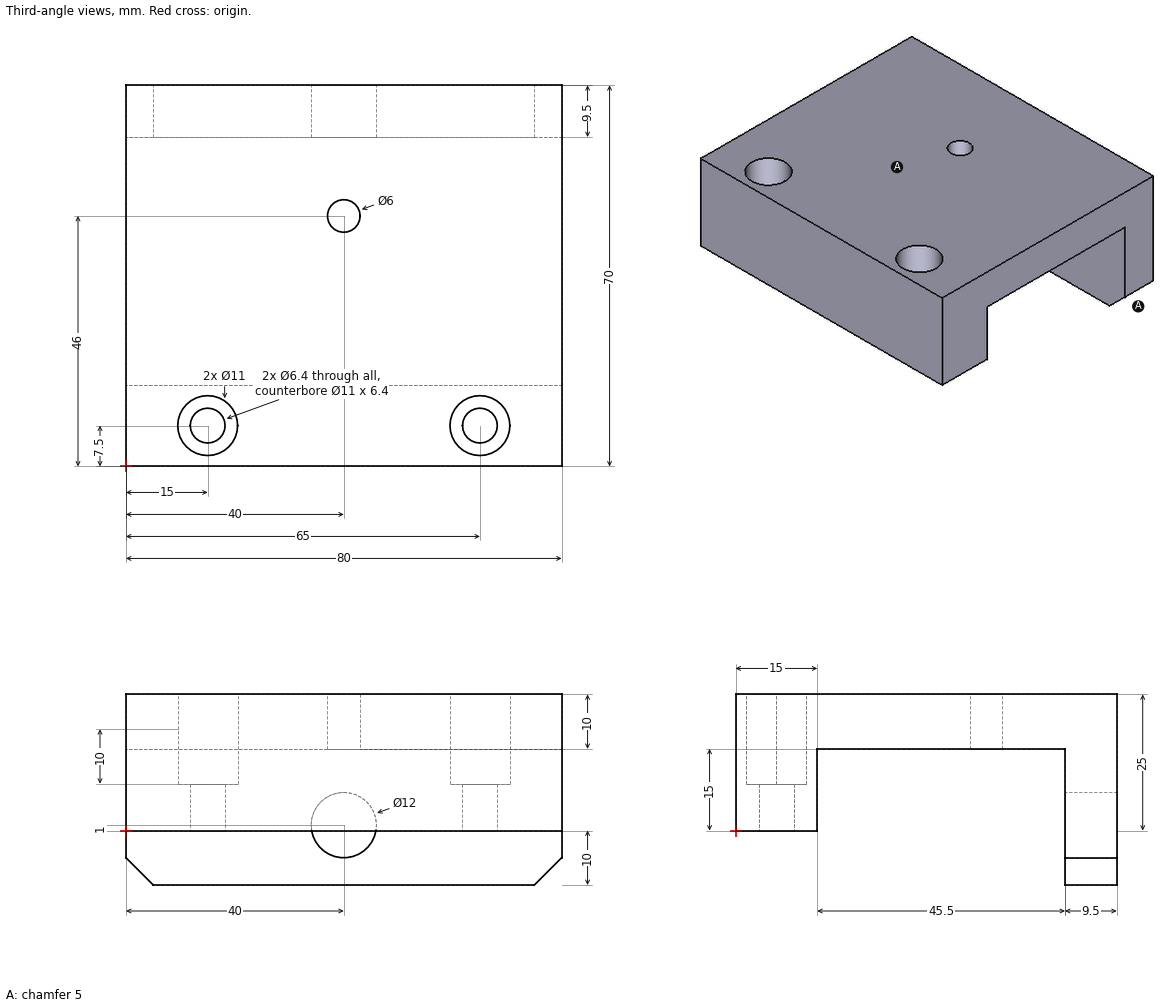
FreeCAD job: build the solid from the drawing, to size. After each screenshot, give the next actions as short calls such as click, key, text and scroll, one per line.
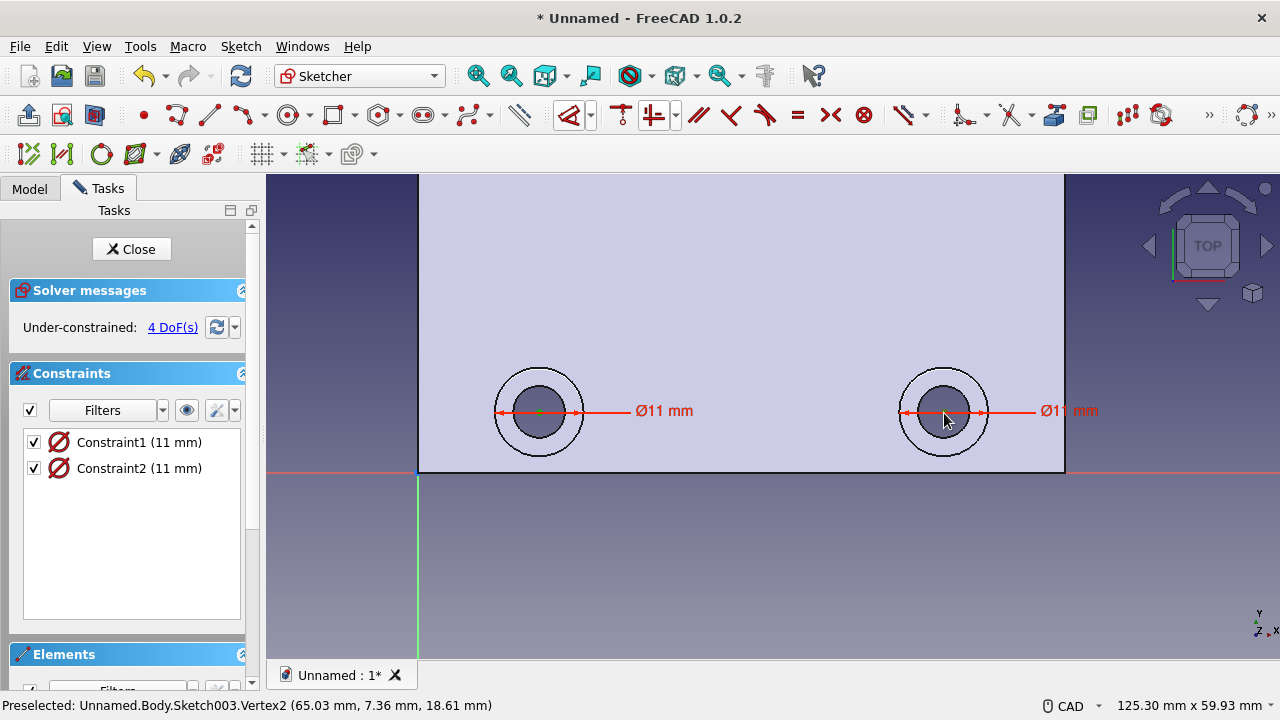
click(676, 116)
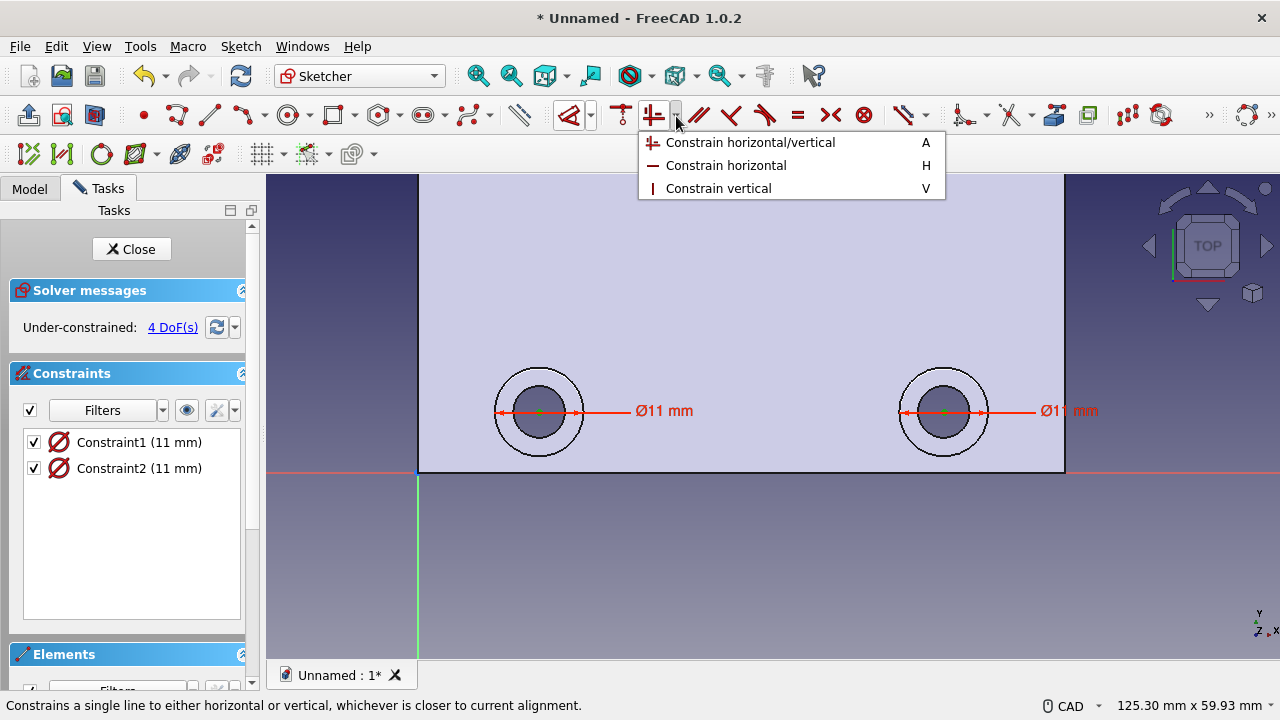
click(792, 166)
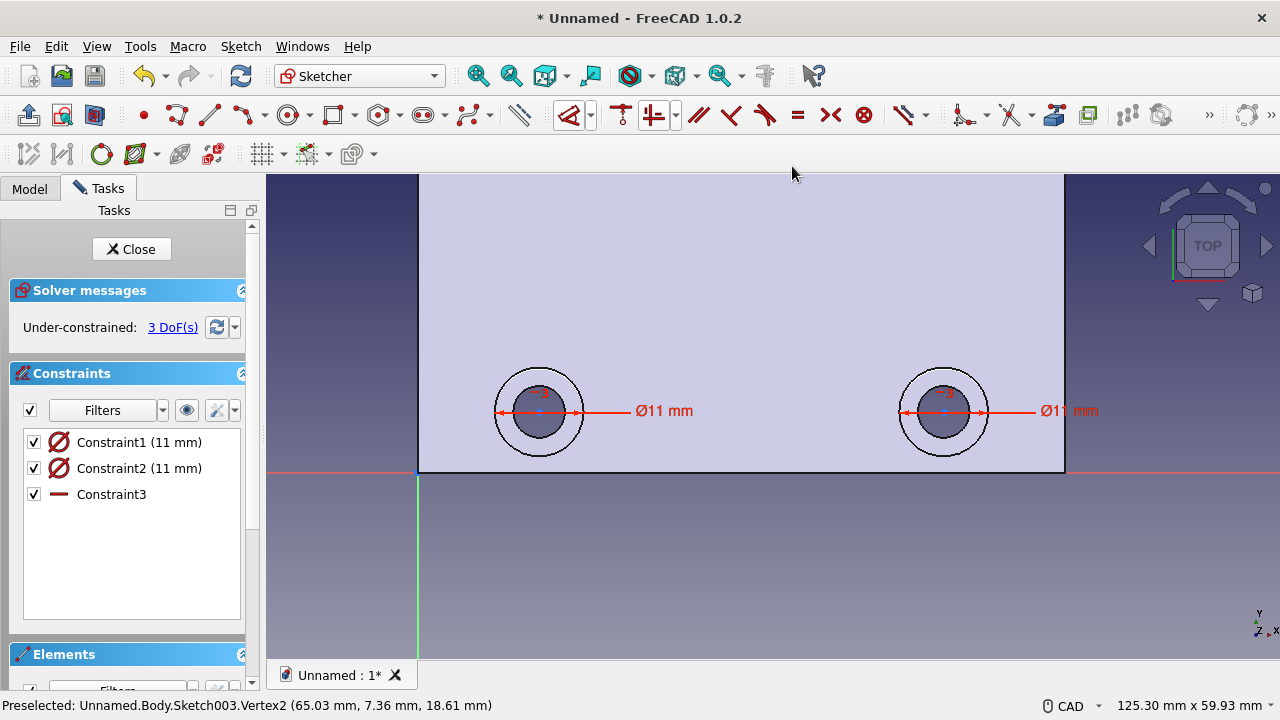
click(539, 413)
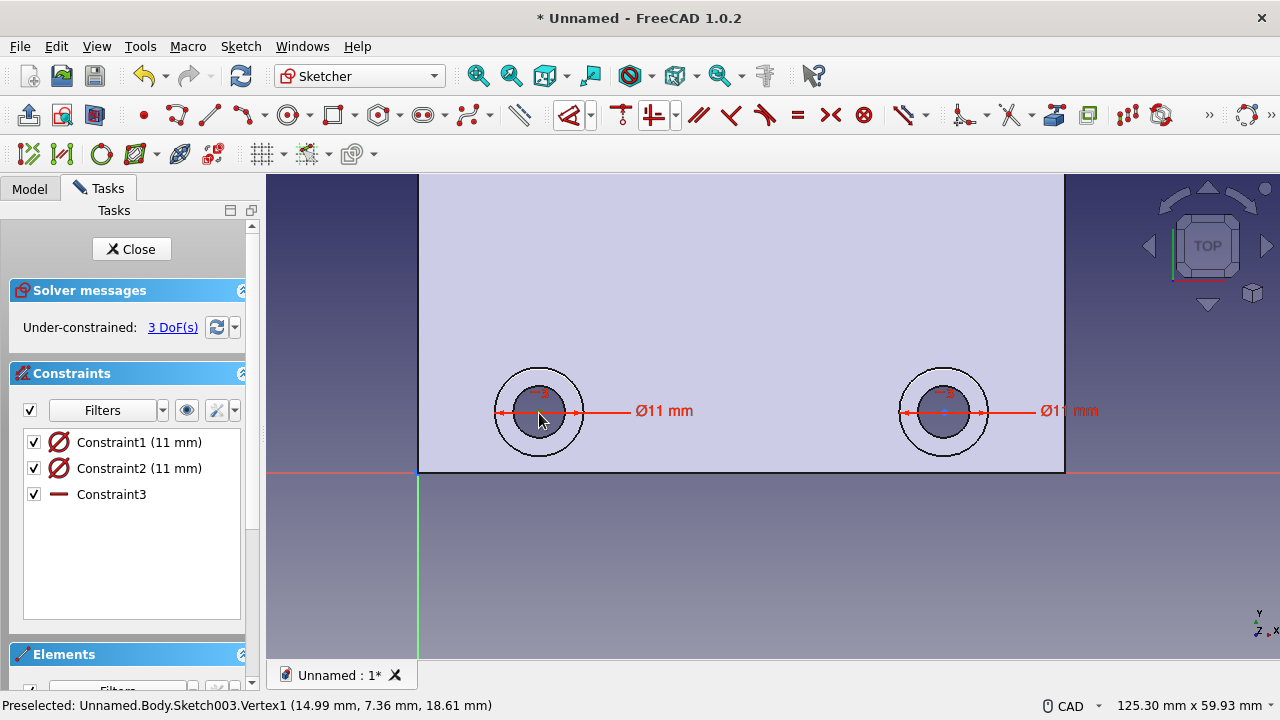
click(590, 116)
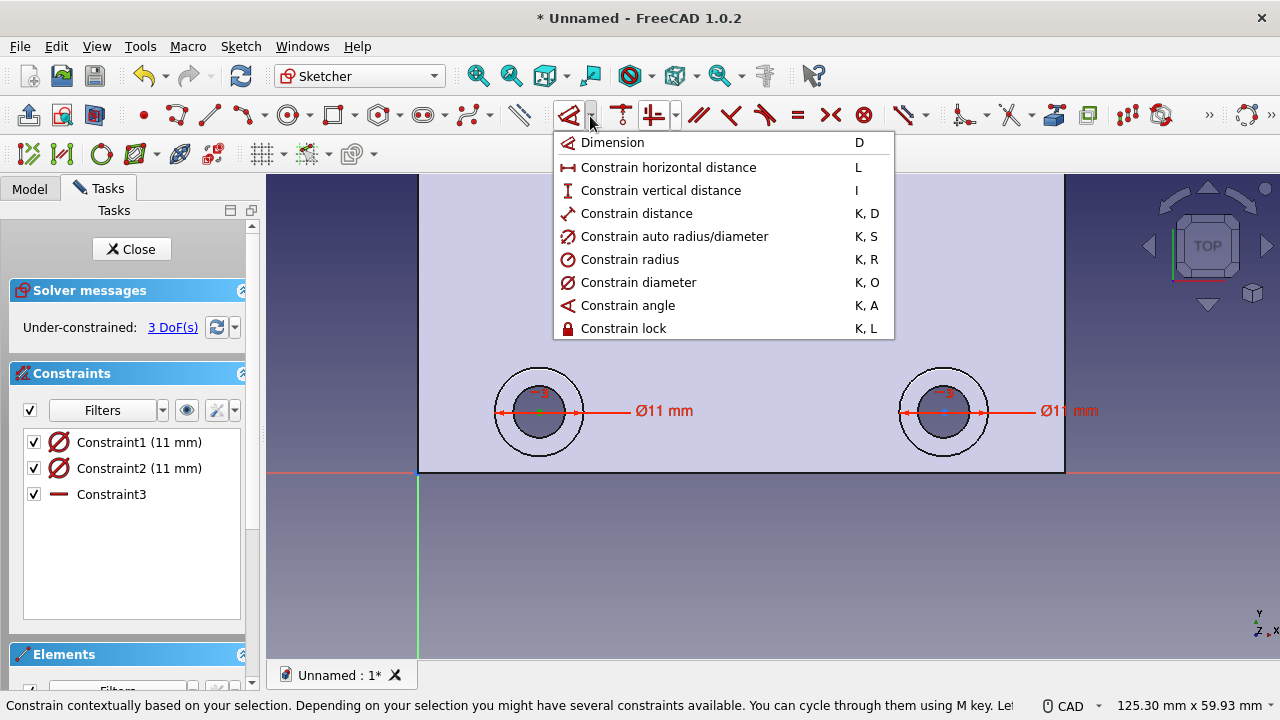
click(724, 168)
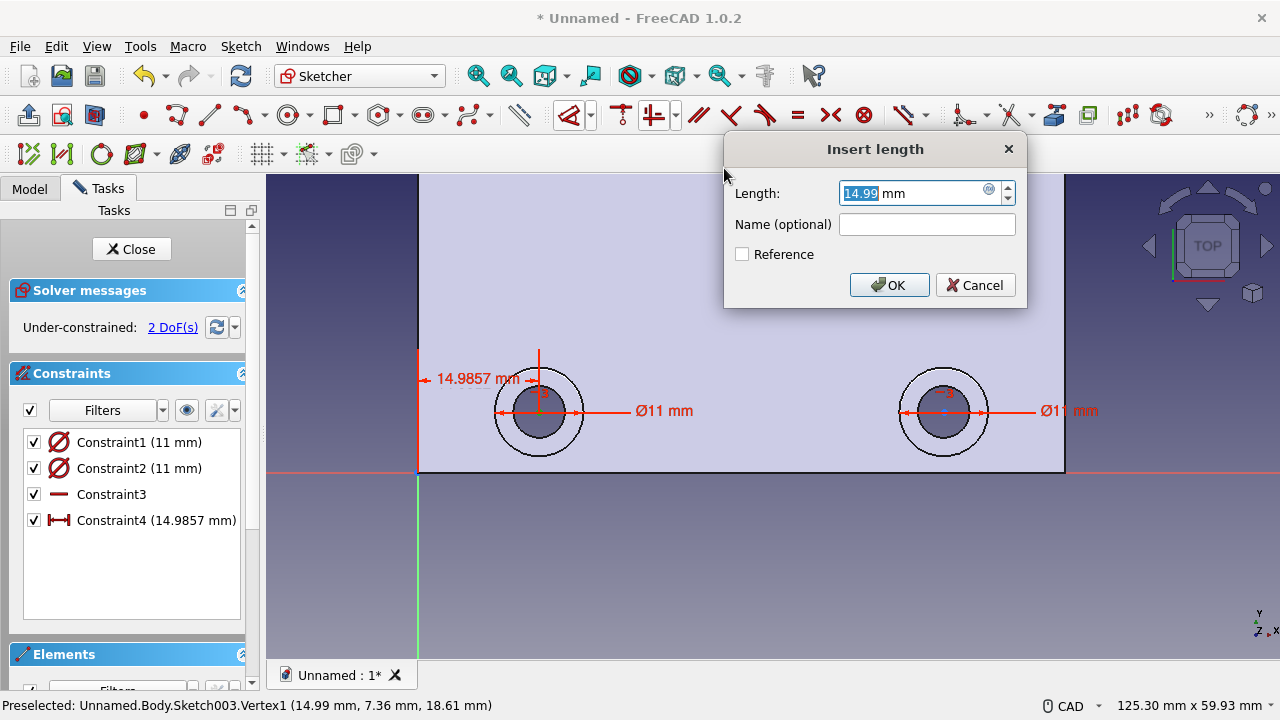
text(15)
key(Return)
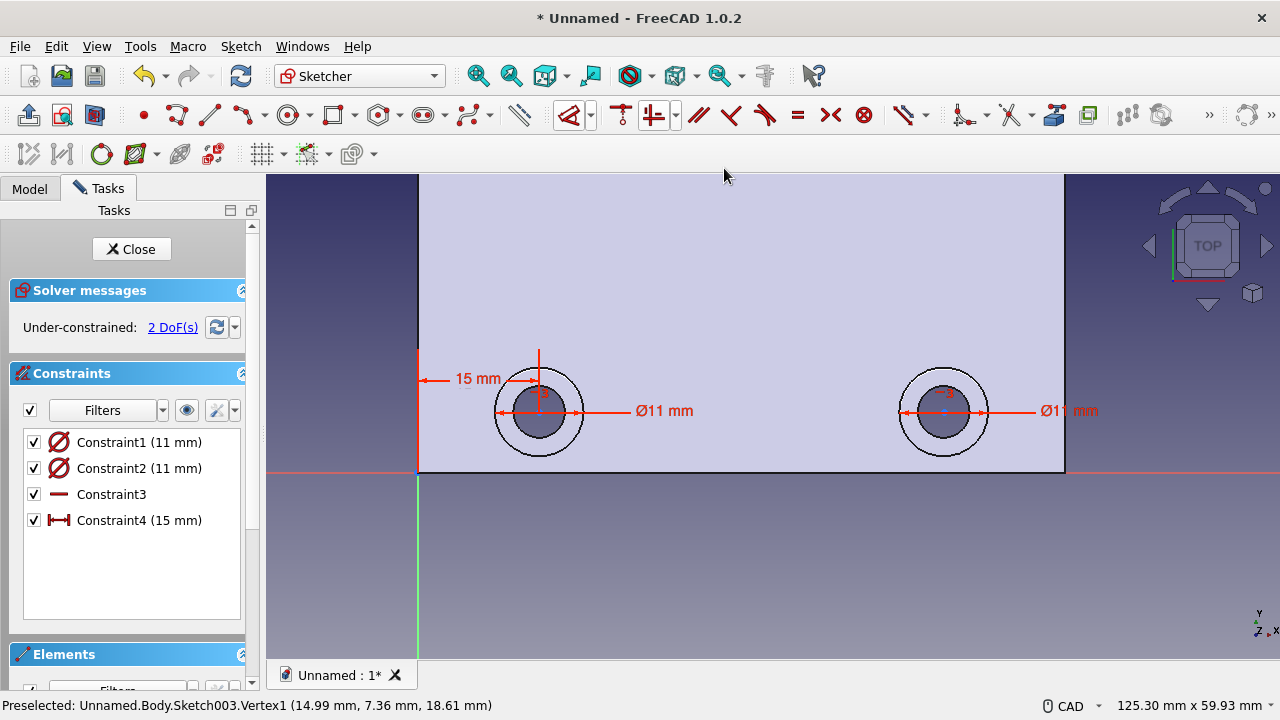
click(944, 413)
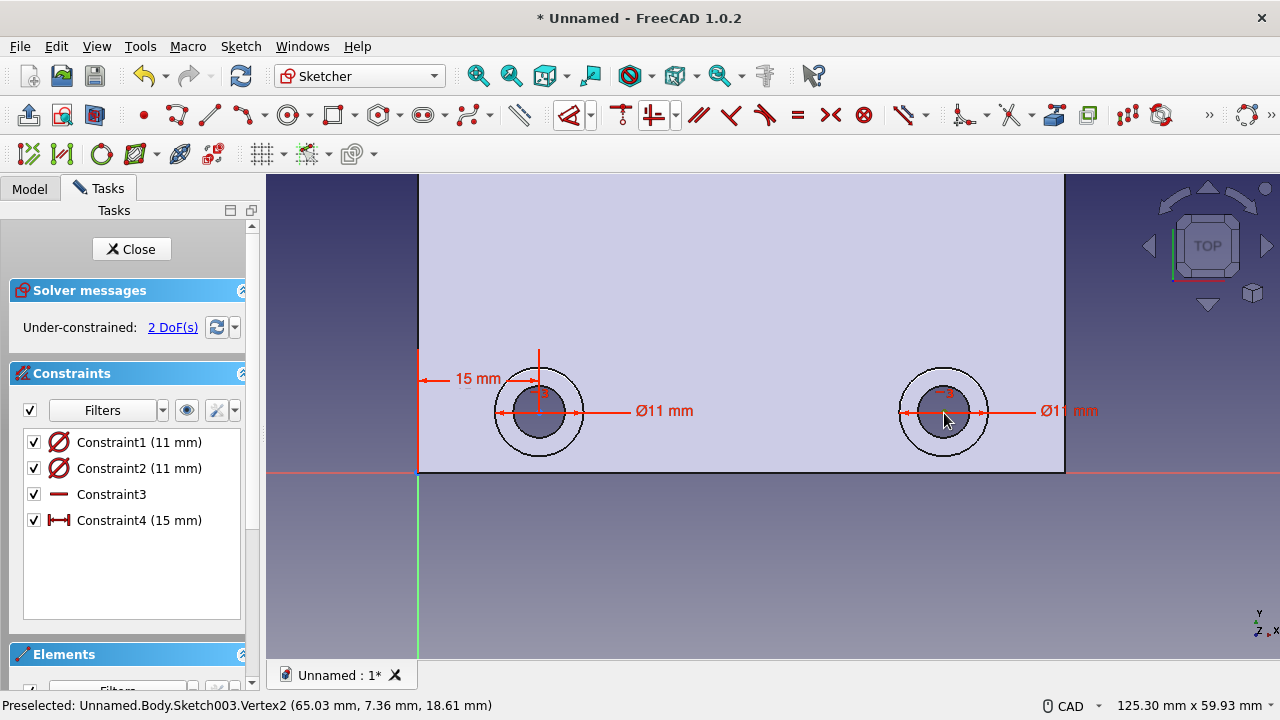
click(590, 116)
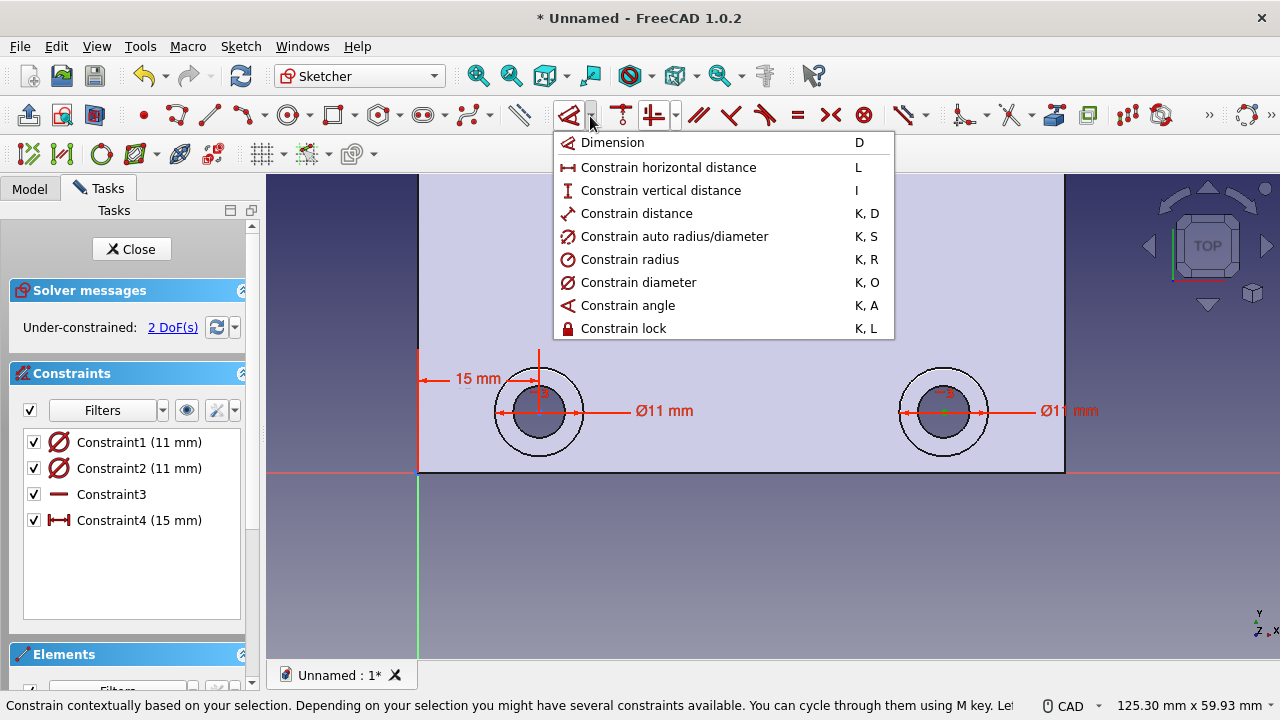
click(724, 168)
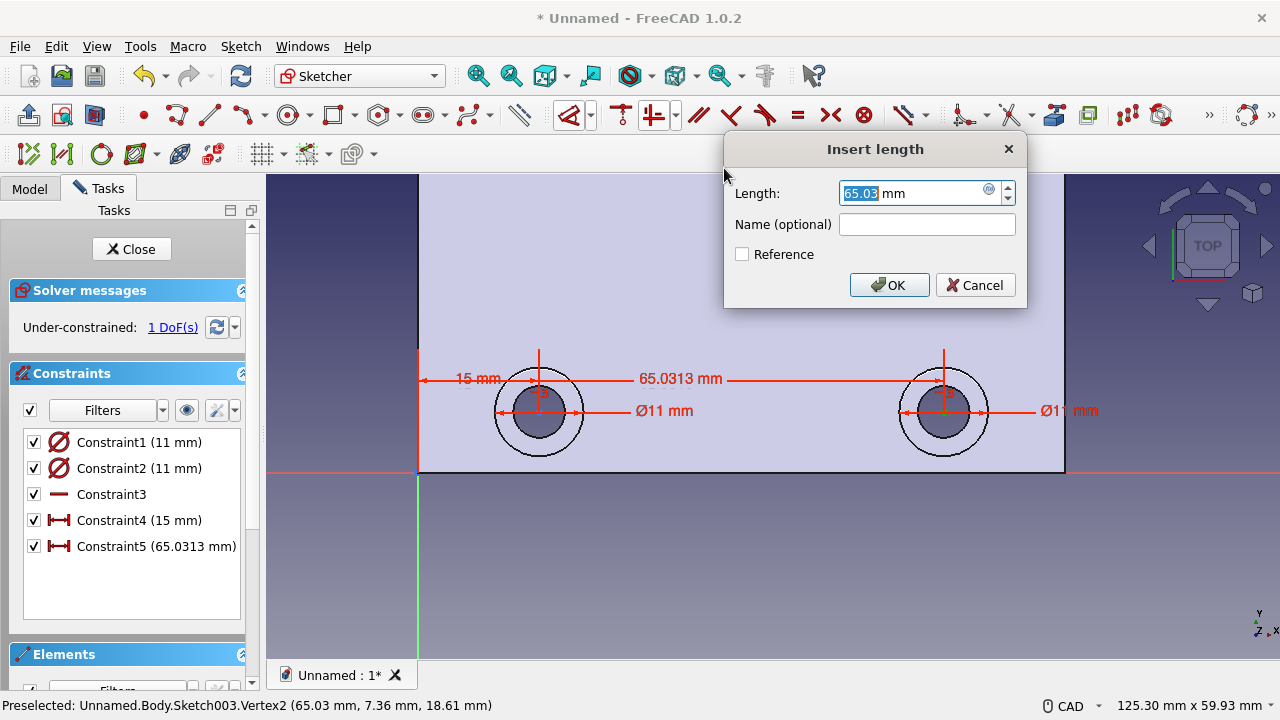
text(65)
key(Return)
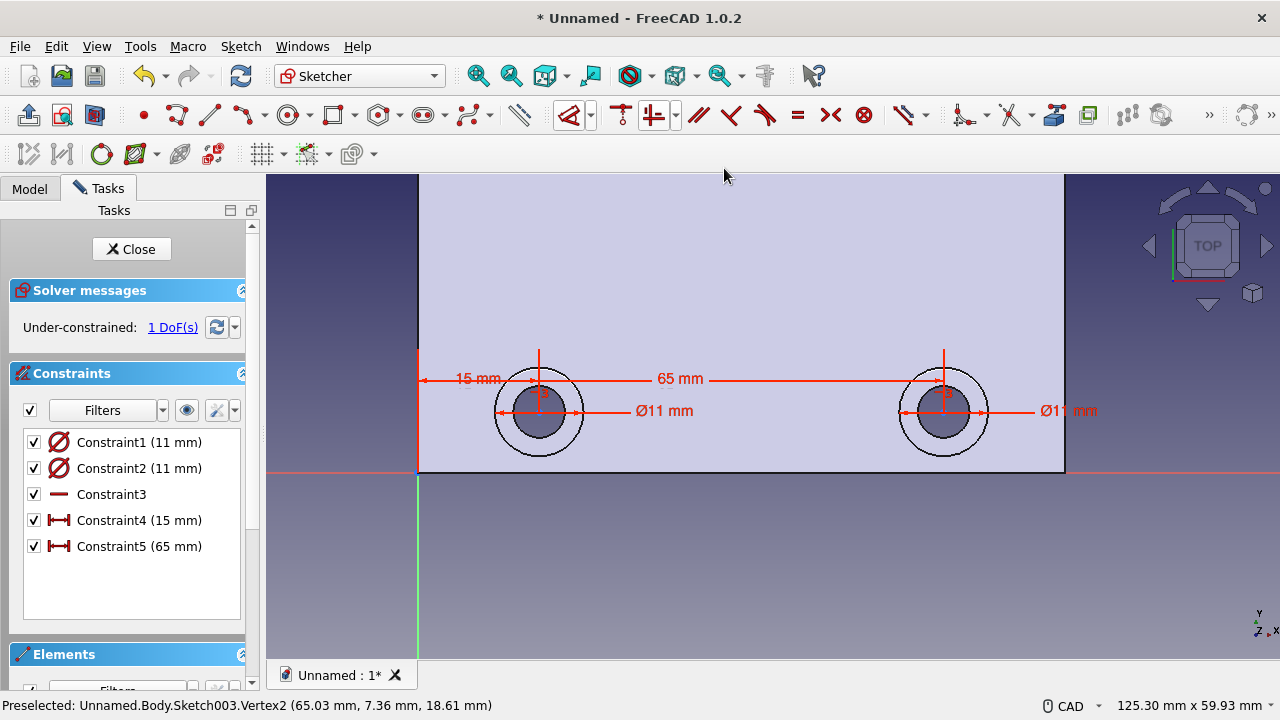
click(539, 413)